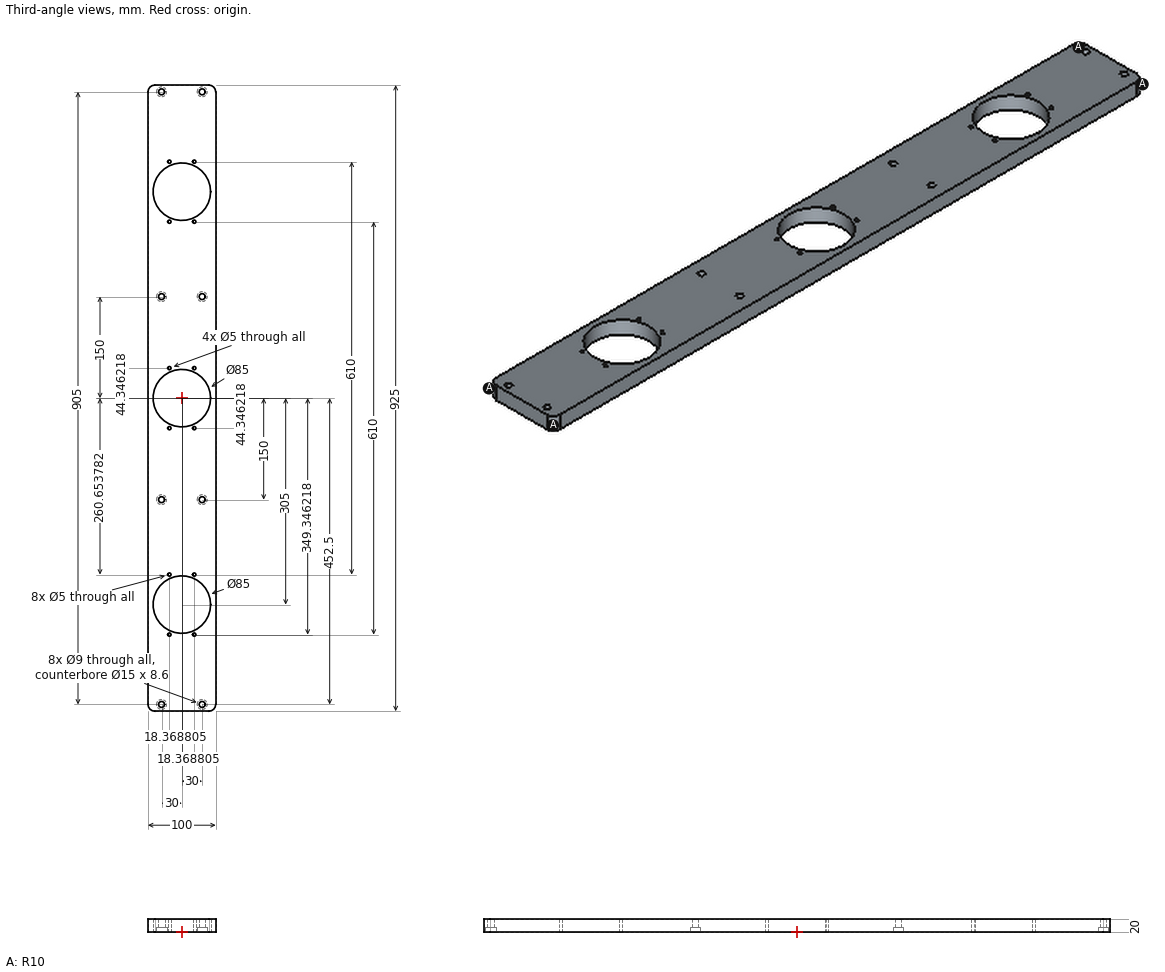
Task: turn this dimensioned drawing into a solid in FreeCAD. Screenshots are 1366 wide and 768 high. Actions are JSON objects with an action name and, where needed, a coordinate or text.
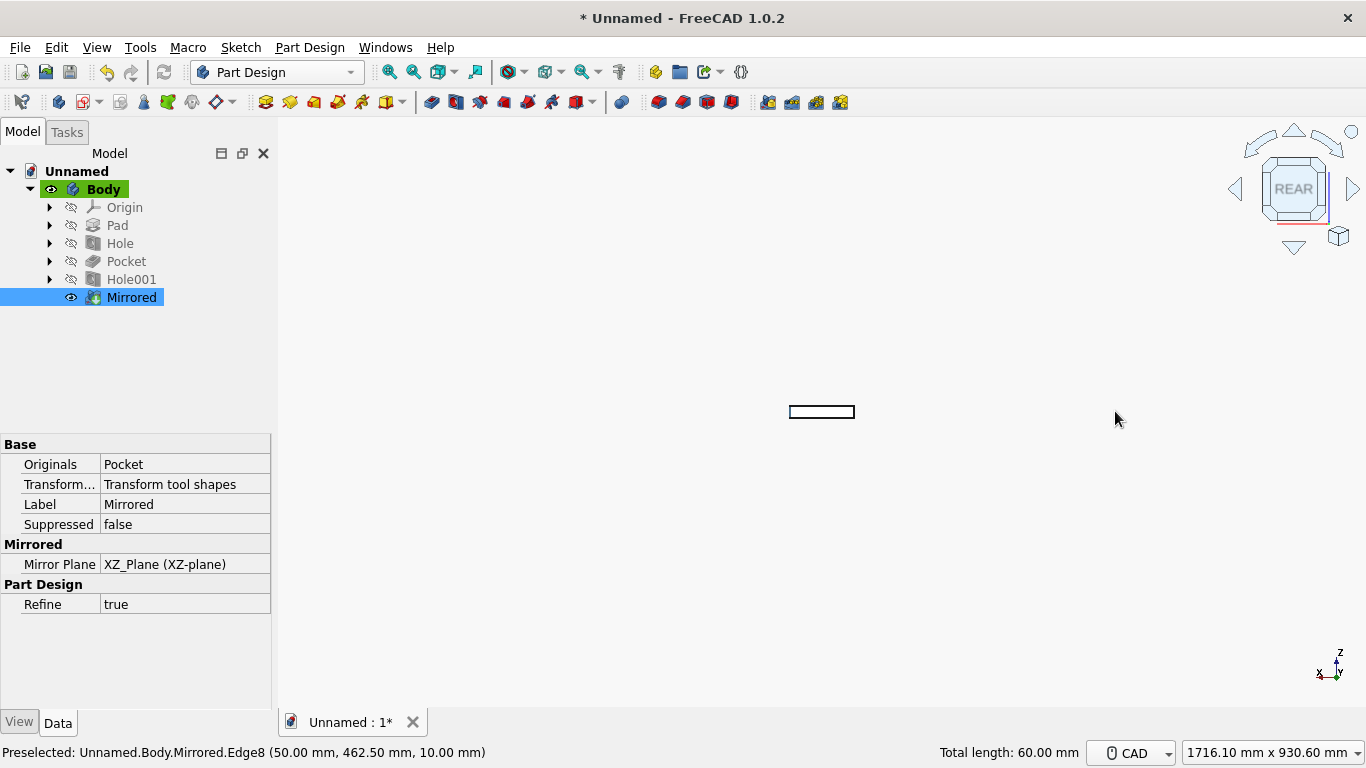
{"action": "key", "text": "v f"}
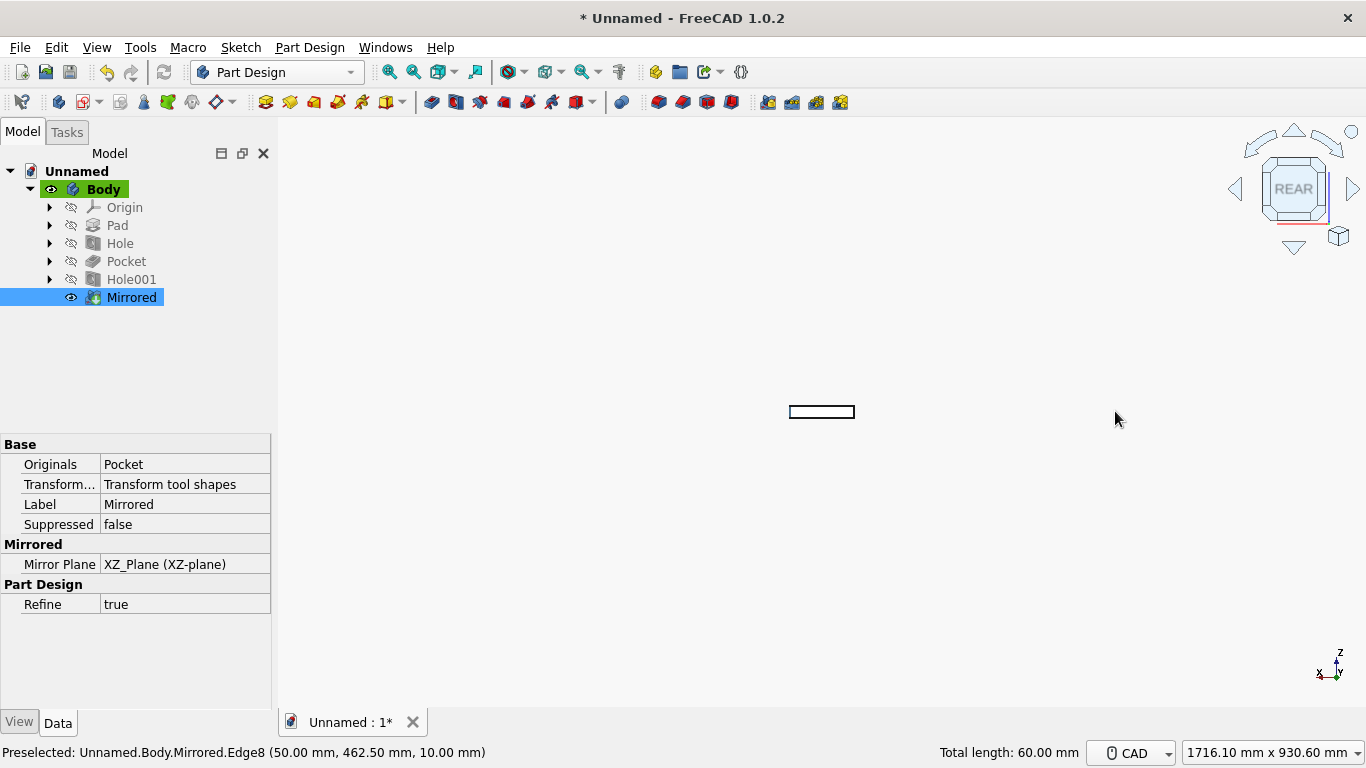
{"action": "left_click", "coordinate": [854, 411], "text": "ctrl"}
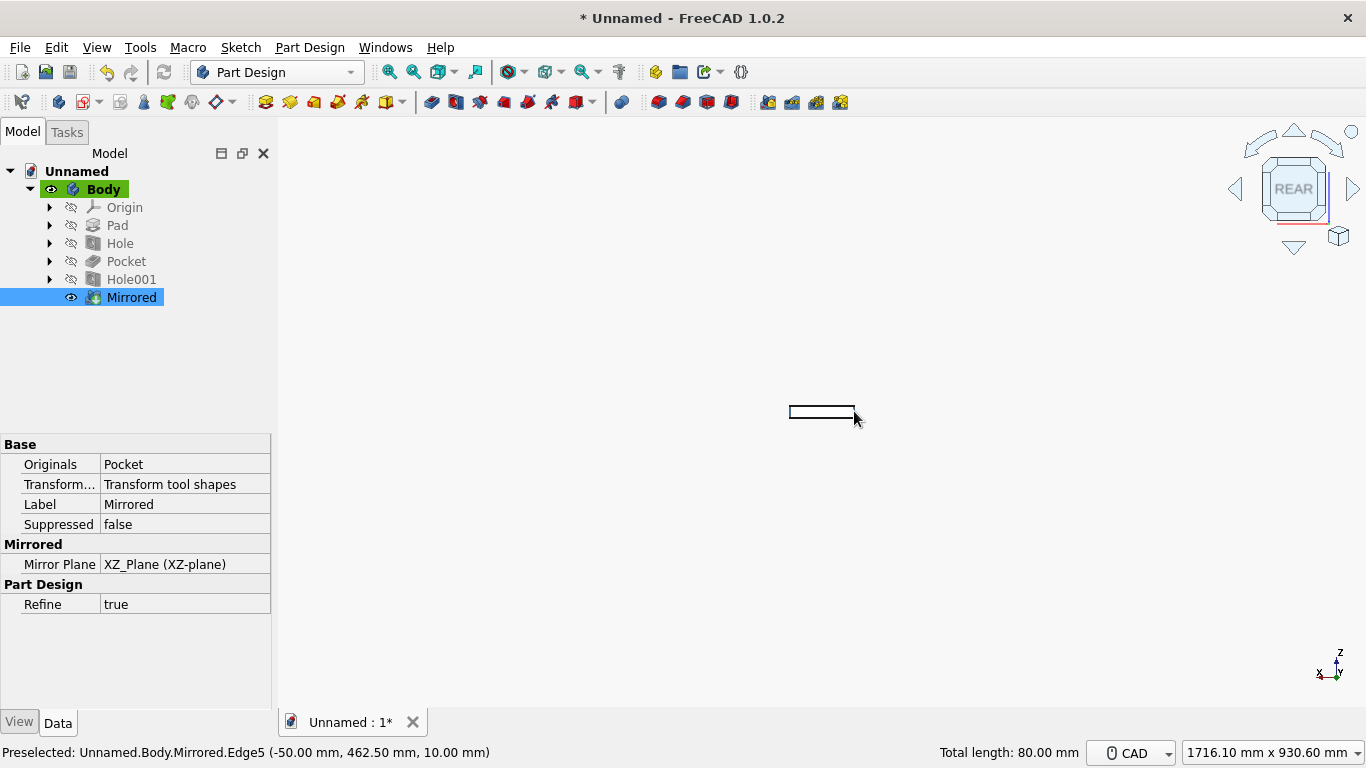
{"action": "left_click", "coordinate": [660, 102]}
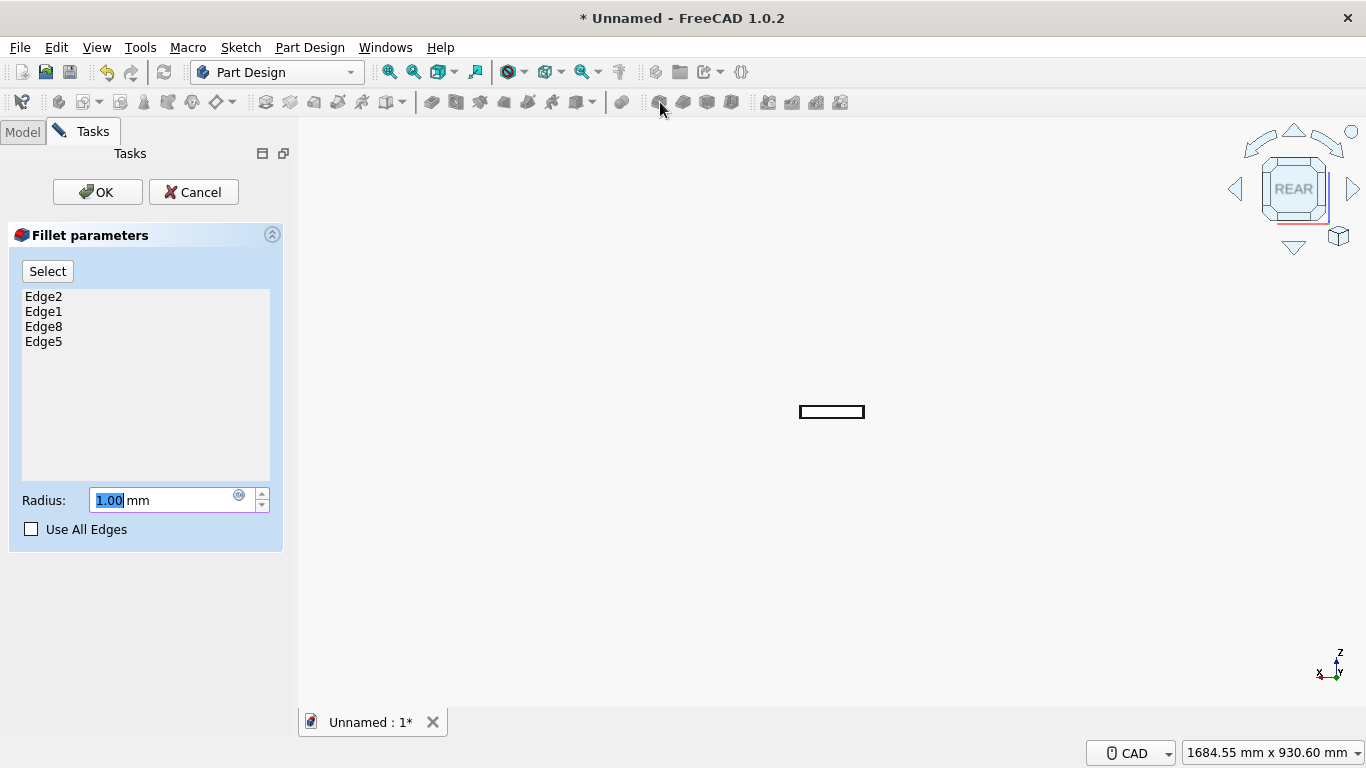
{"action": "type", "text": "10"}
{"action": "key", "text": "Tab"}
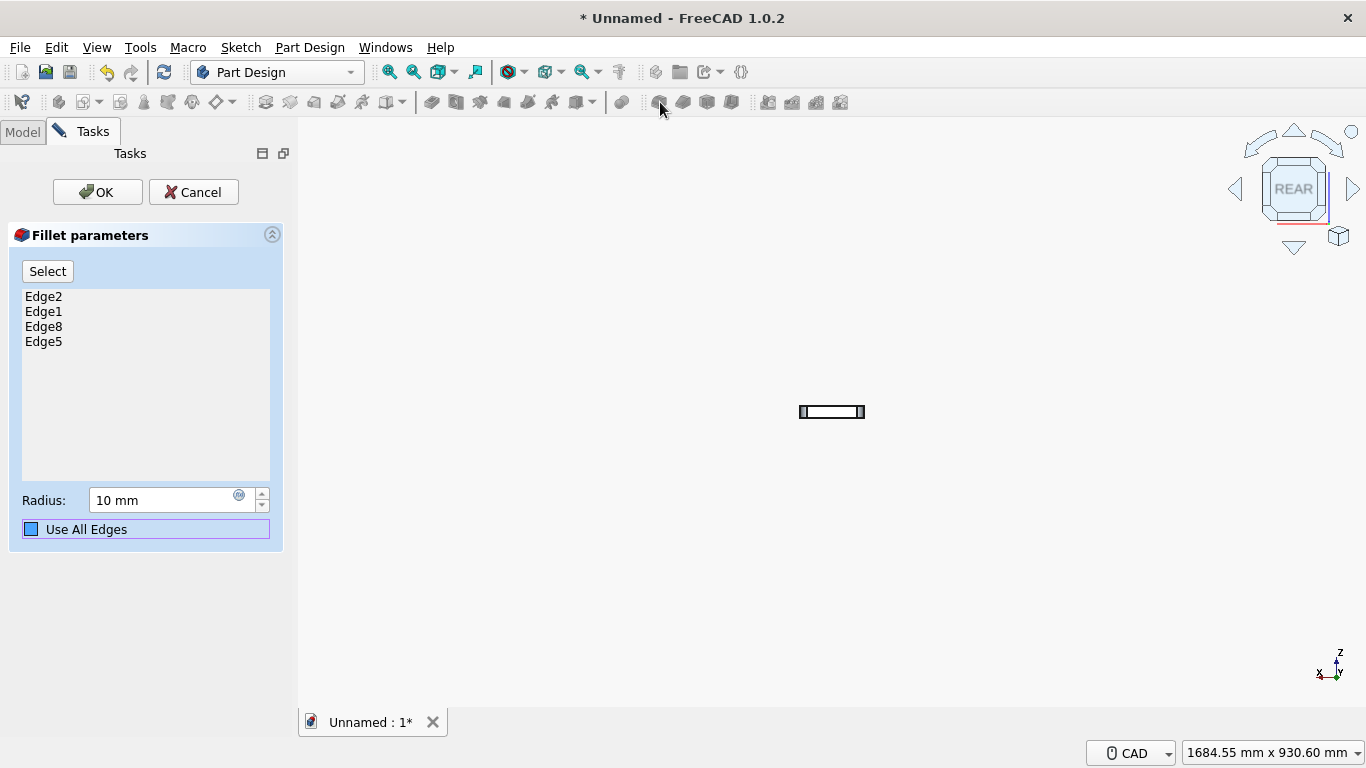
{"action": "left_click", "coordinate": [98, 192]}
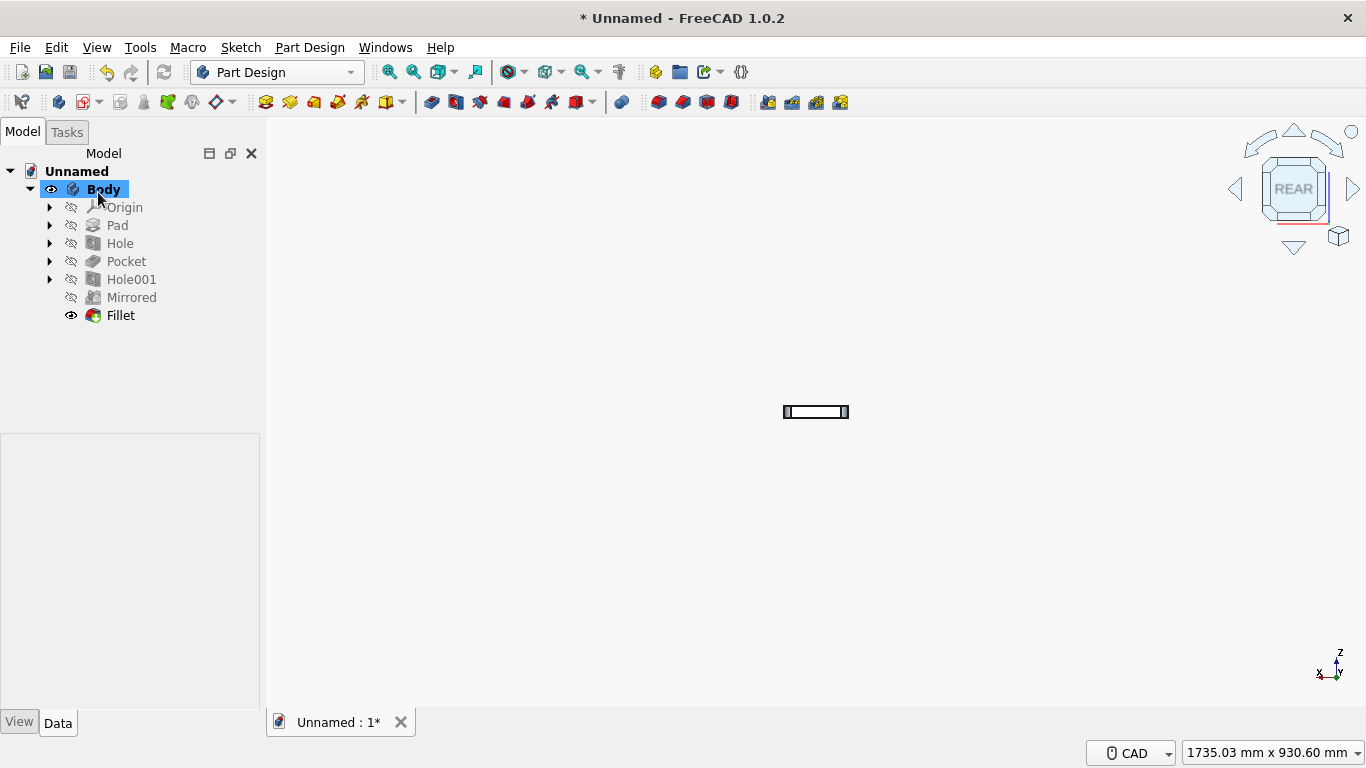
{"action": "left_click", "coordinate": [390, 72]}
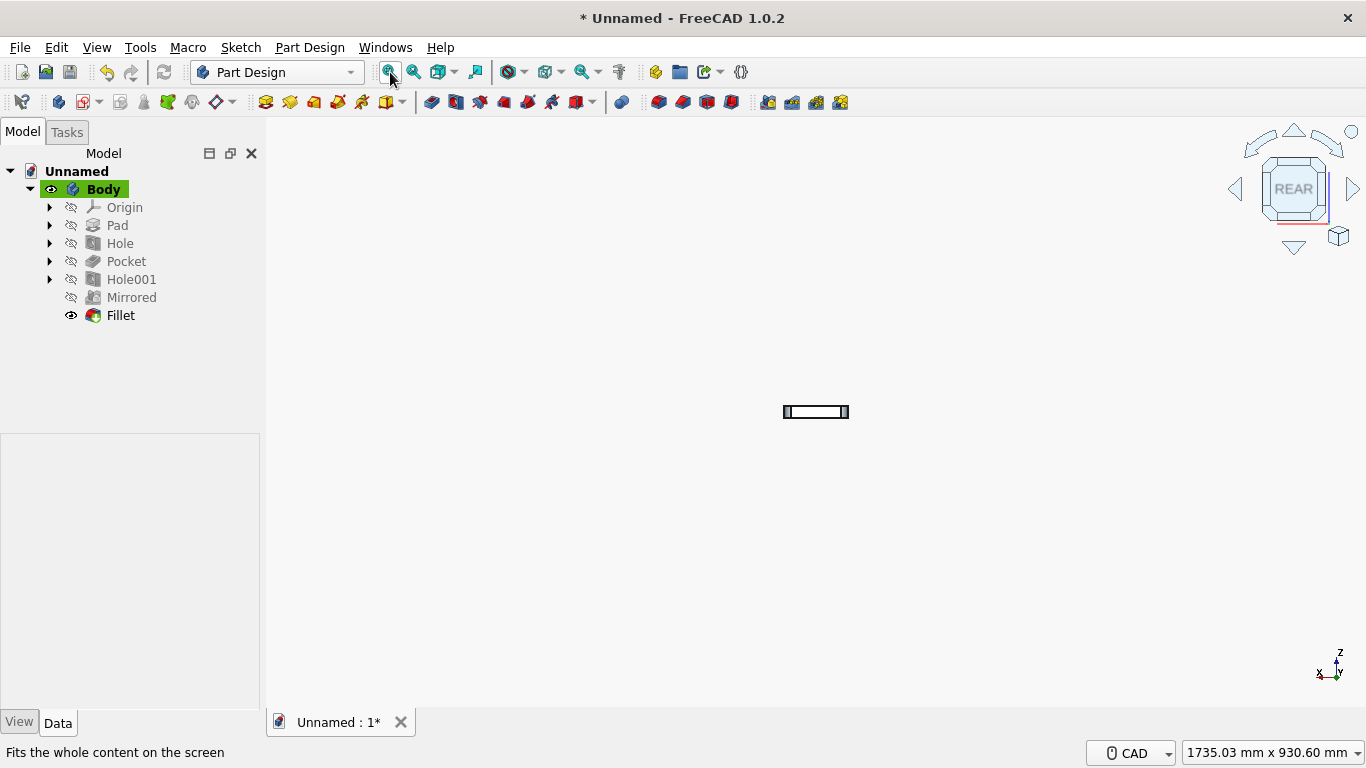
{"action": "key", "text": "0"}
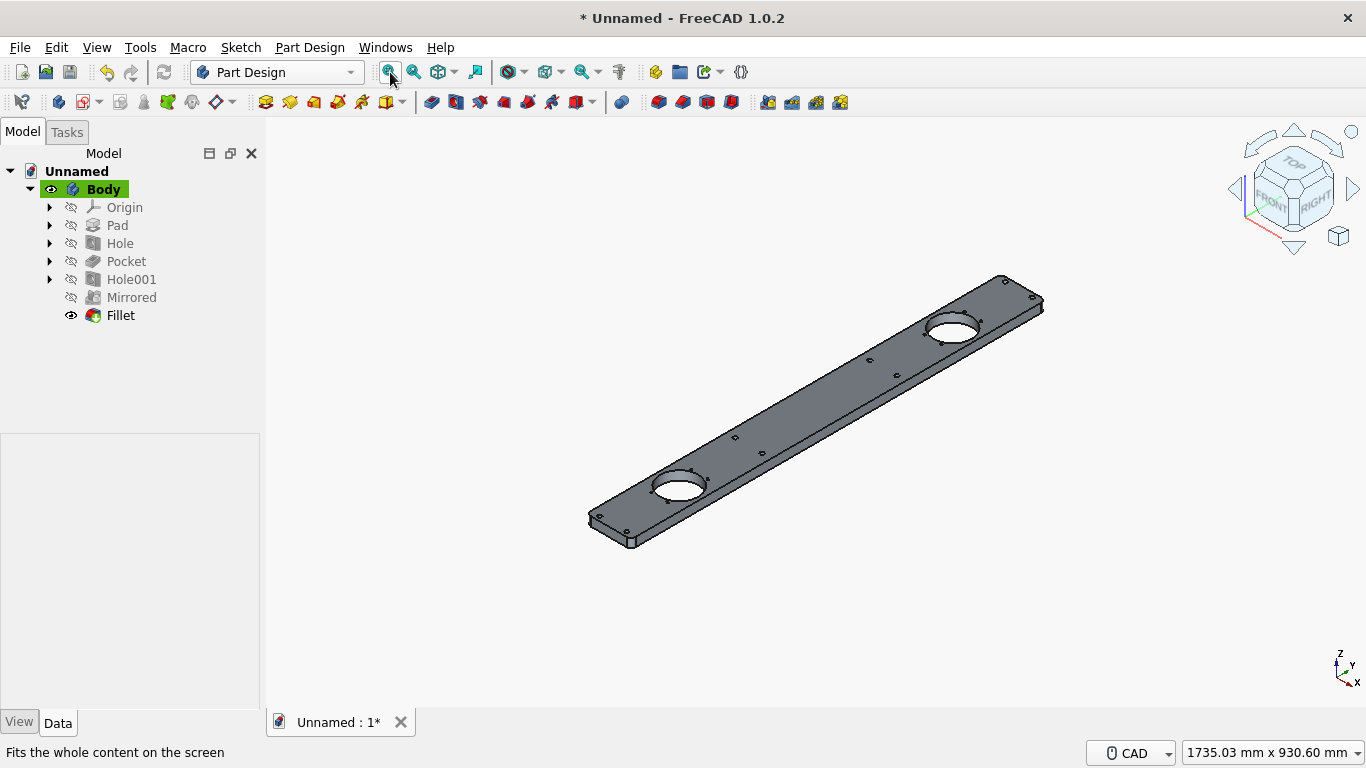
{"action": "left_click", "coordinate": [816, 406]}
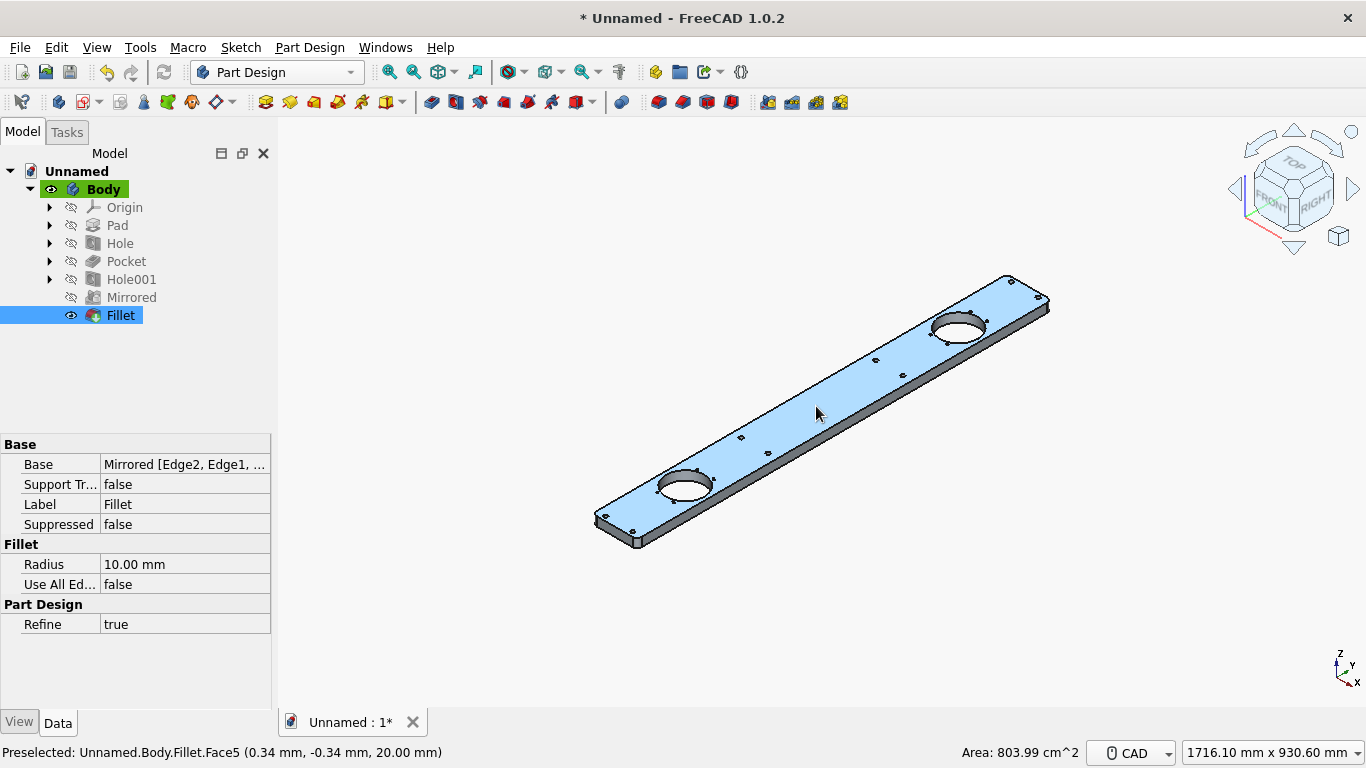
{"action": "left_click", "coordinate": [84, 102]}